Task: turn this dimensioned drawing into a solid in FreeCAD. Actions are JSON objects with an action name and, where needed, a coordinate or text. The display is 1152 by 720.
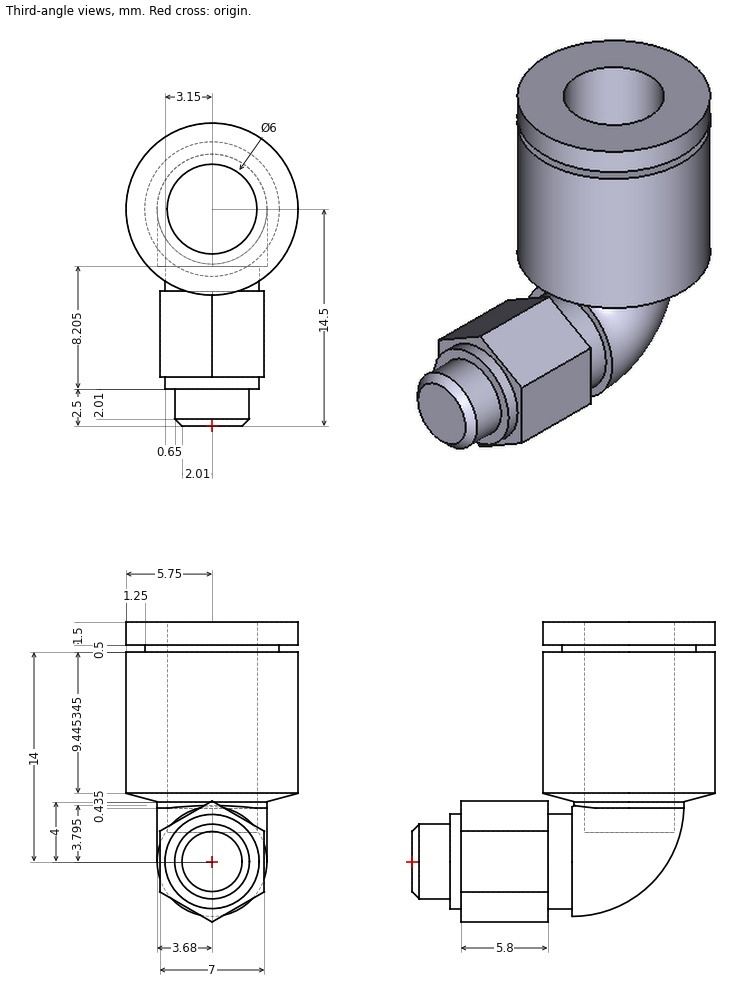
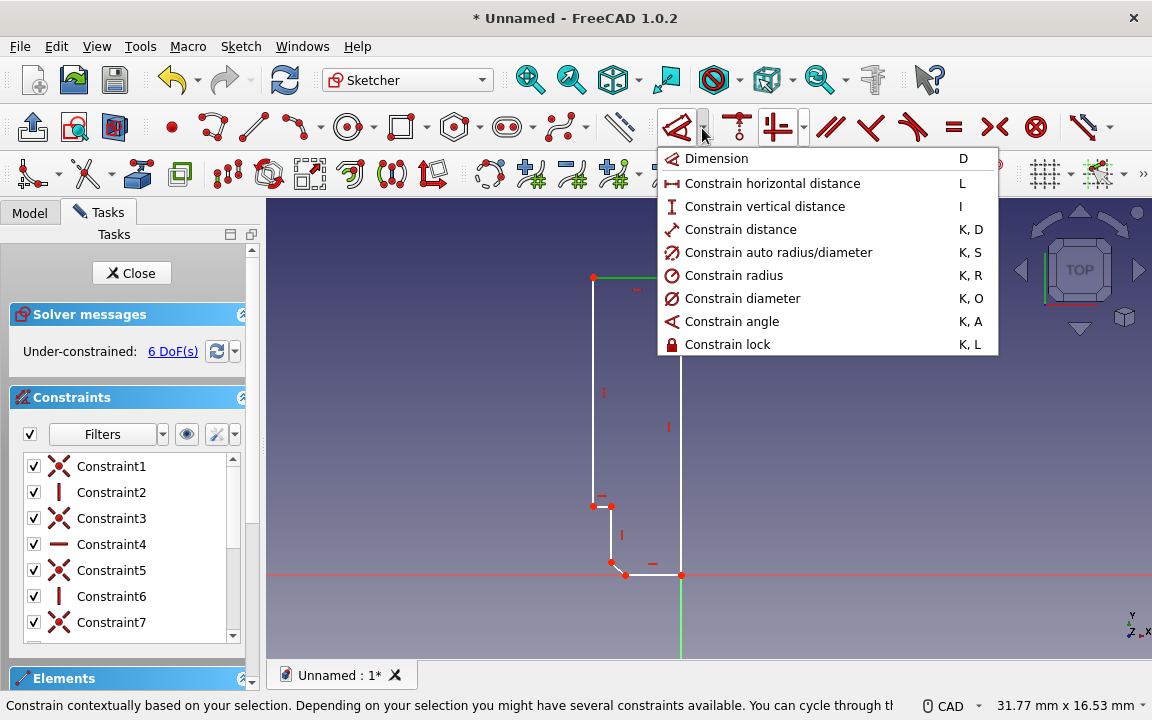
{"action": "left_click", "coordinate": [828, 184]}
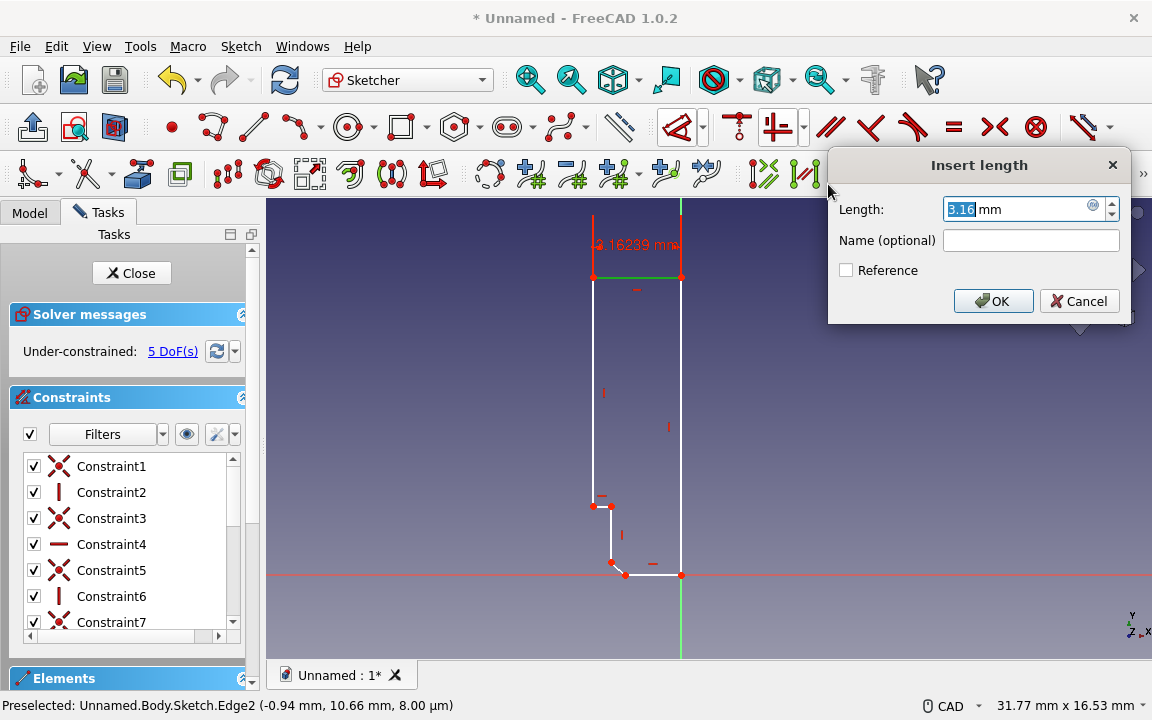
{"action": "type", "text": "3.15"}
{"action": "key", "text": "Return"}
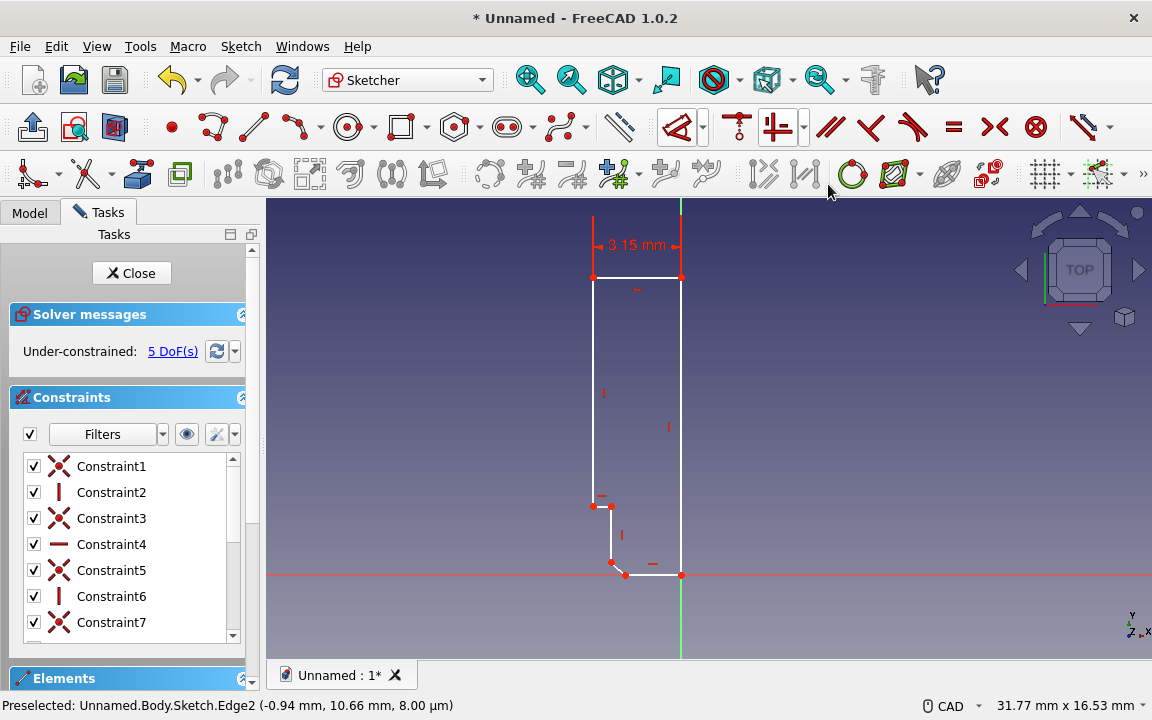
{"action": "scroll", "coordinate": [602, 507], "scroll_direction": "up", "scroll_amount": 4}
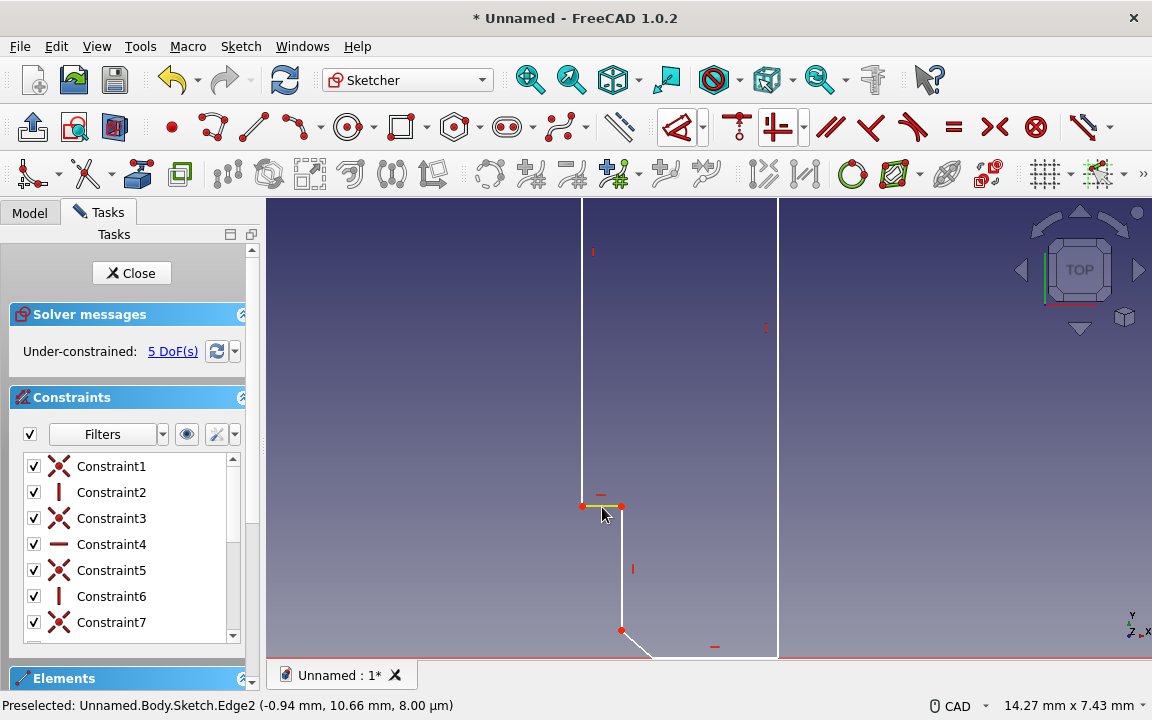
{"action": "left_click", "coordinate": [602, 506]}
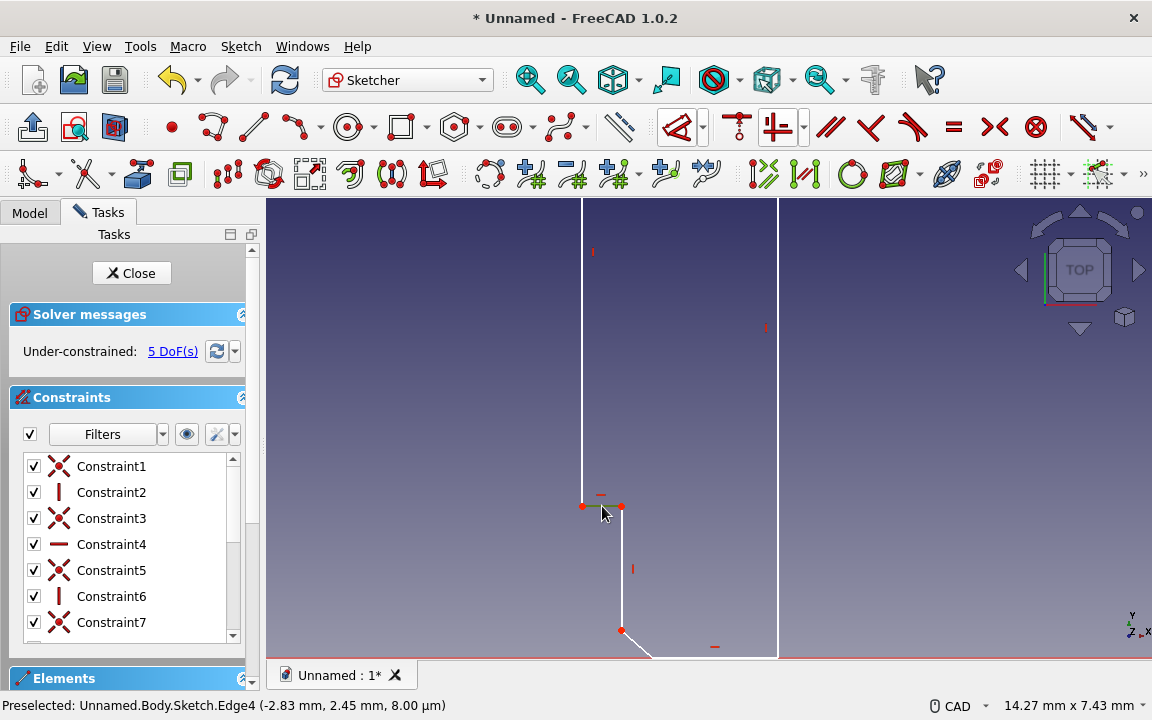
{"action": "left_click", "coordinate": [702, 128]}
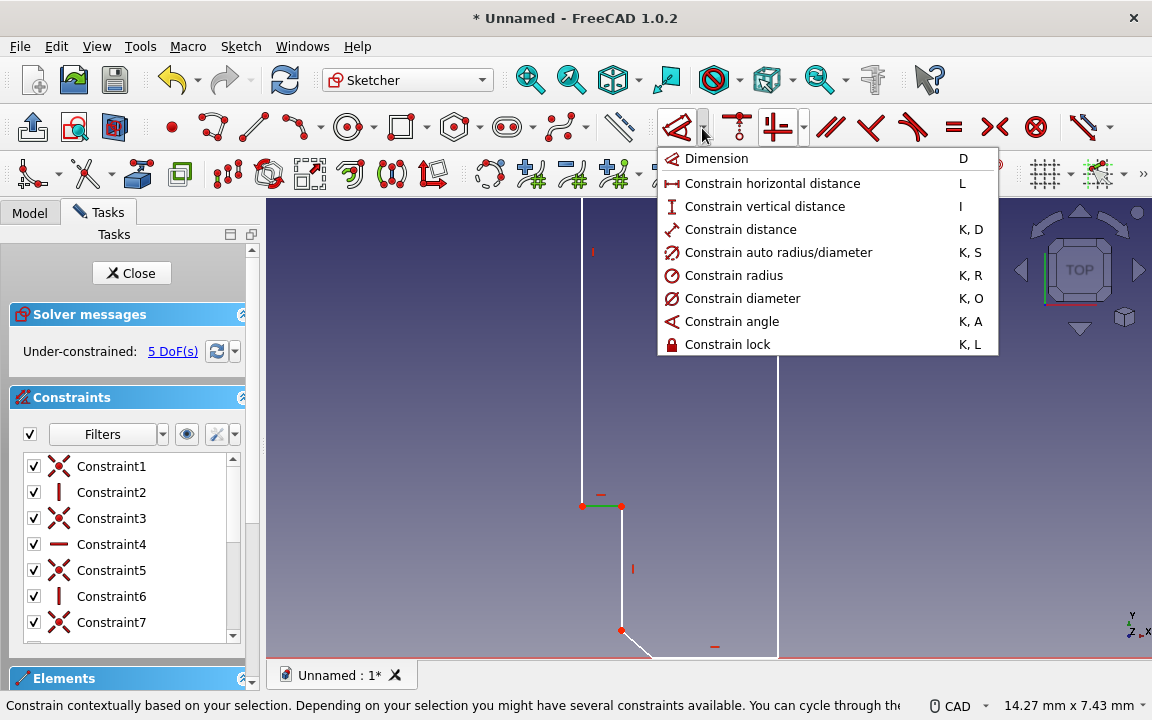
{"action": "left_click", "coordinate": [828, 184]}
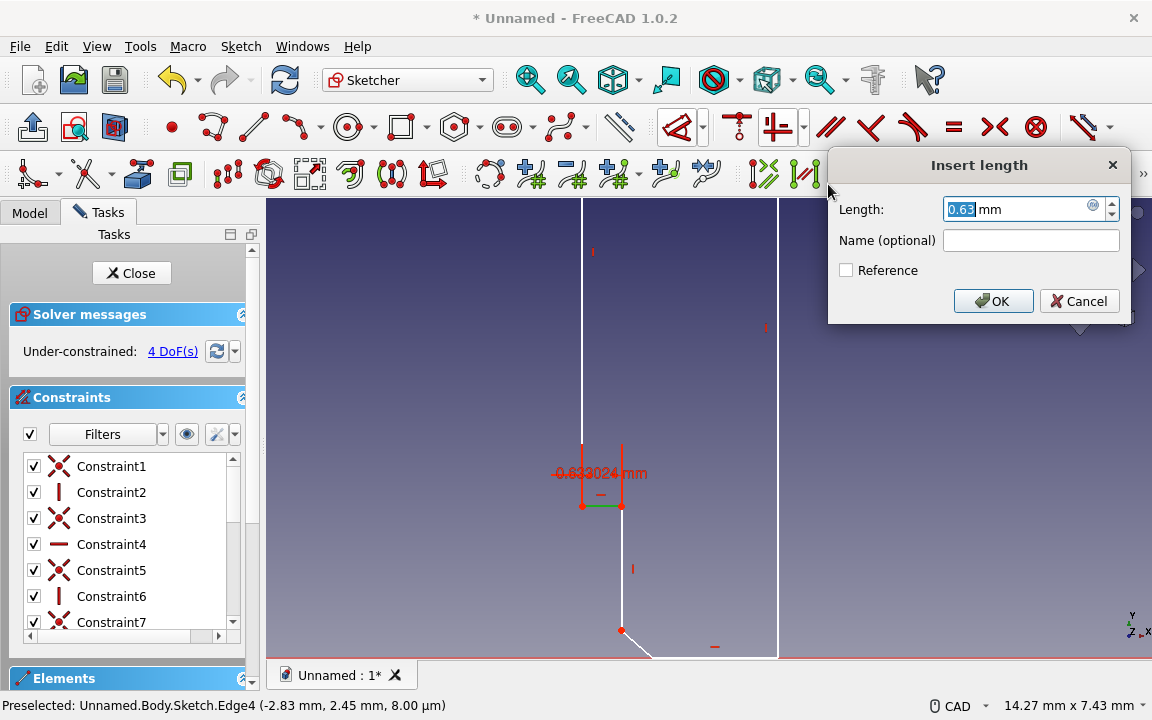
{"action": "type", "text": "0.65"}
{"action": "key", "text": "Return"}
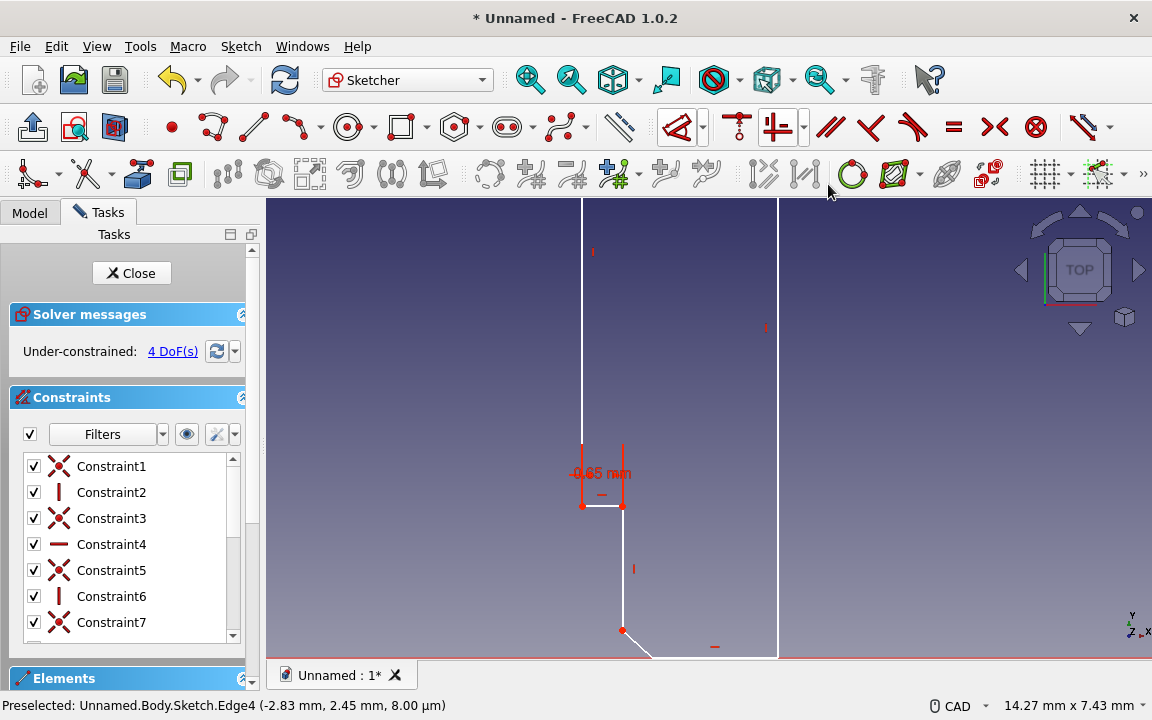
{"action": "left_click", "coordinate": [623, 544]}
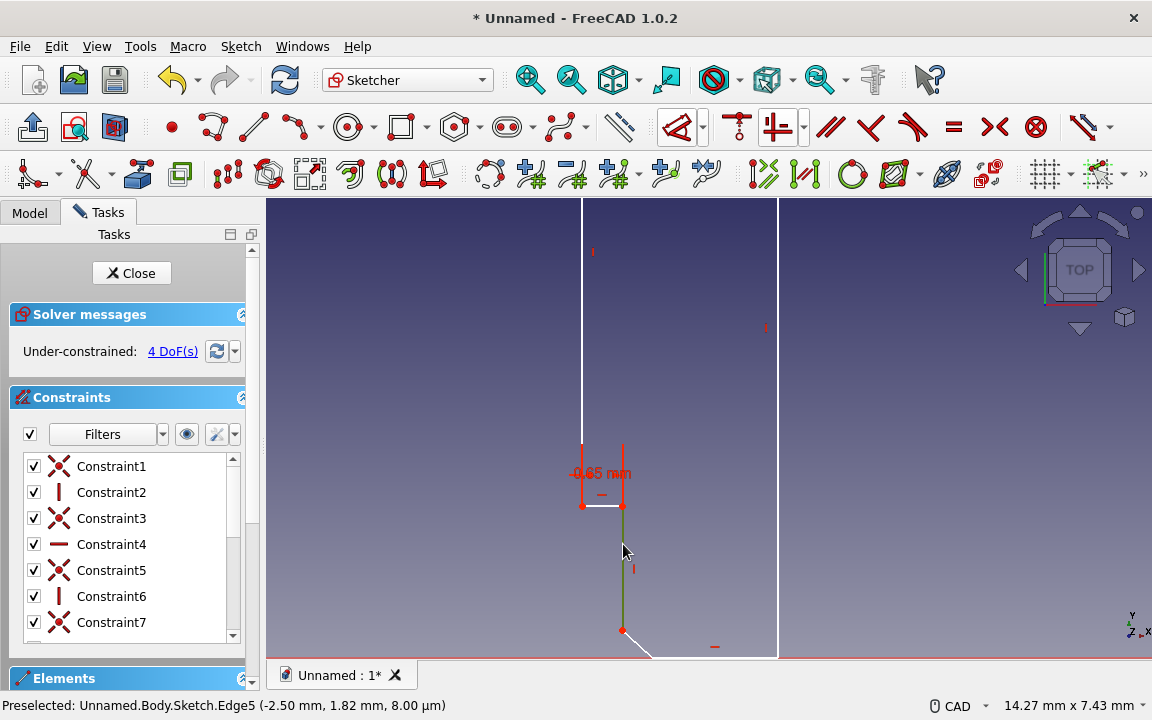
{"action": "key", "text": "i"}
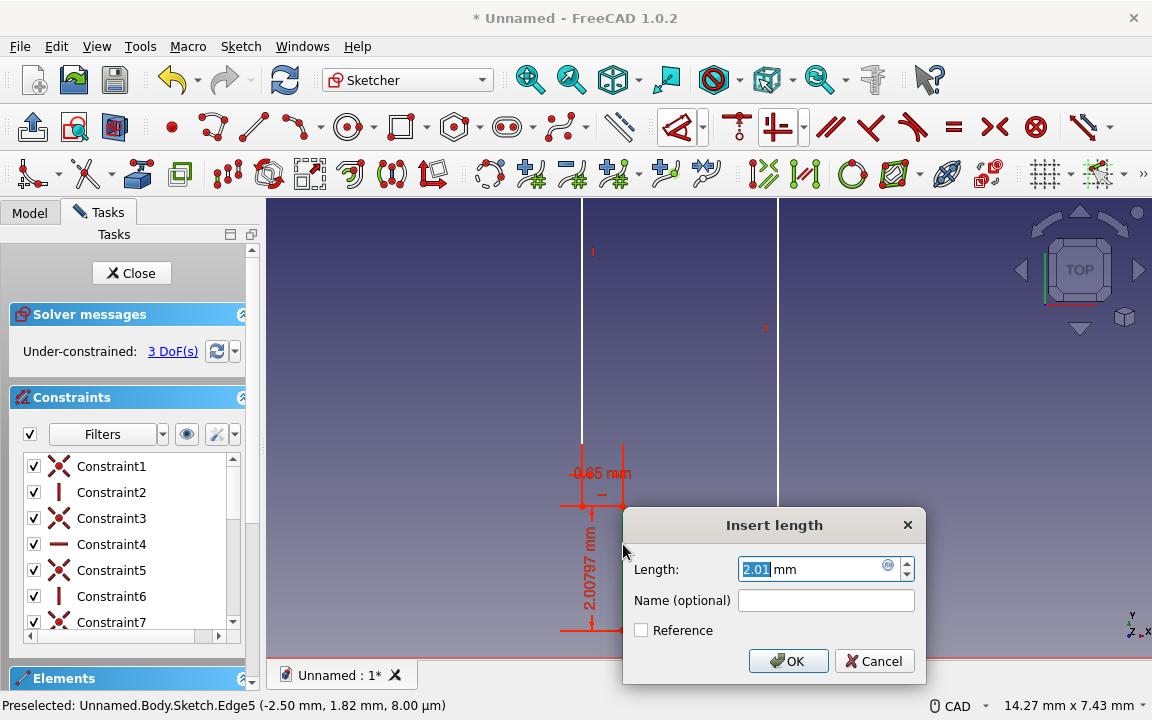
{"action": "type", "text": "2.01"}
{"action": "key", "text": "Return"}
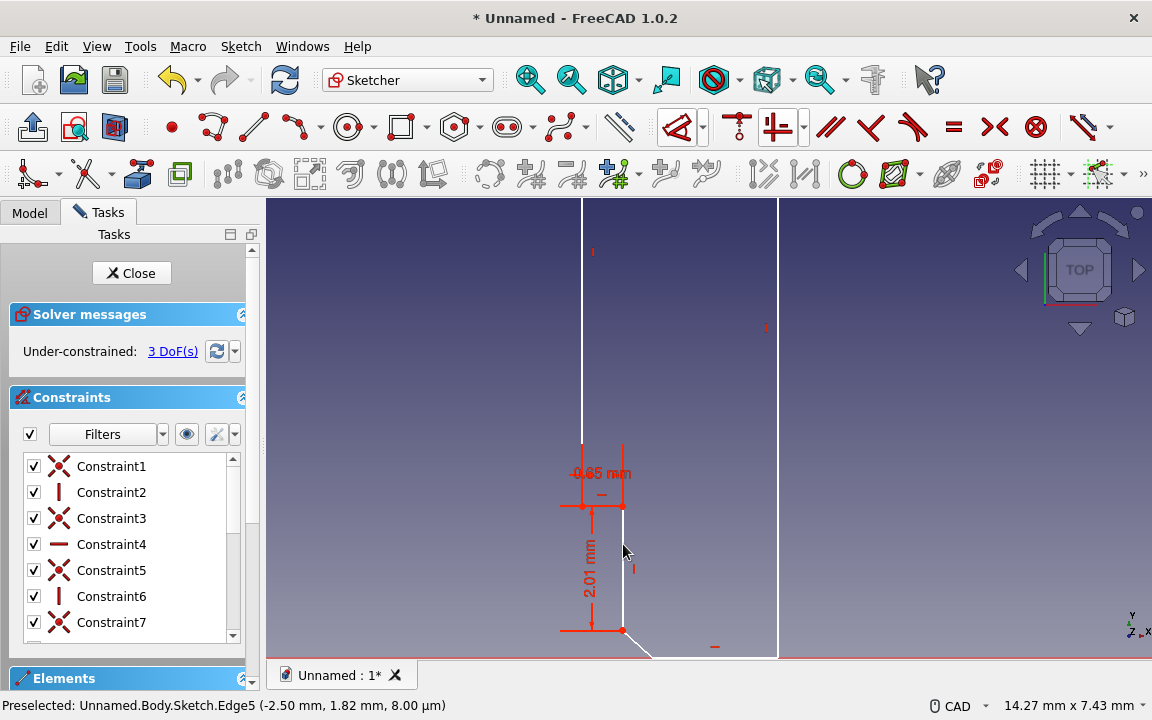
{"action": "scroll", "coordinate": [608, 512], "scroll_direction": "down", "scroll_amount": 4}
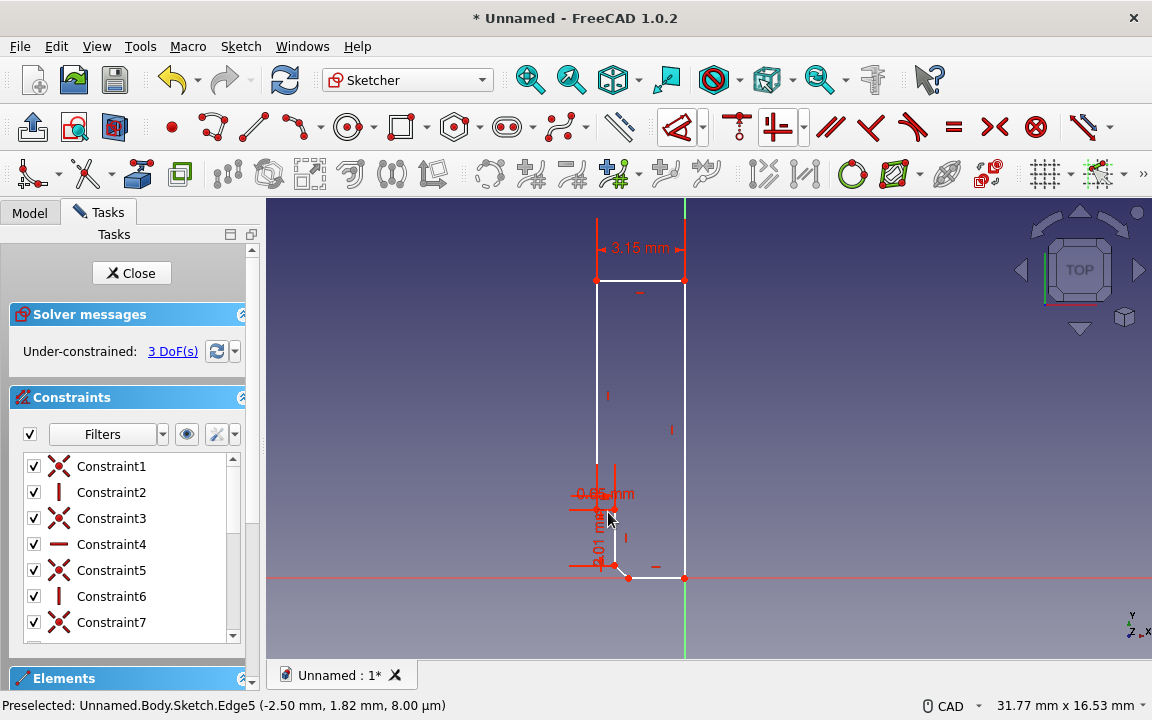
{"action": "left_click", "coordinate": [645, 578]}